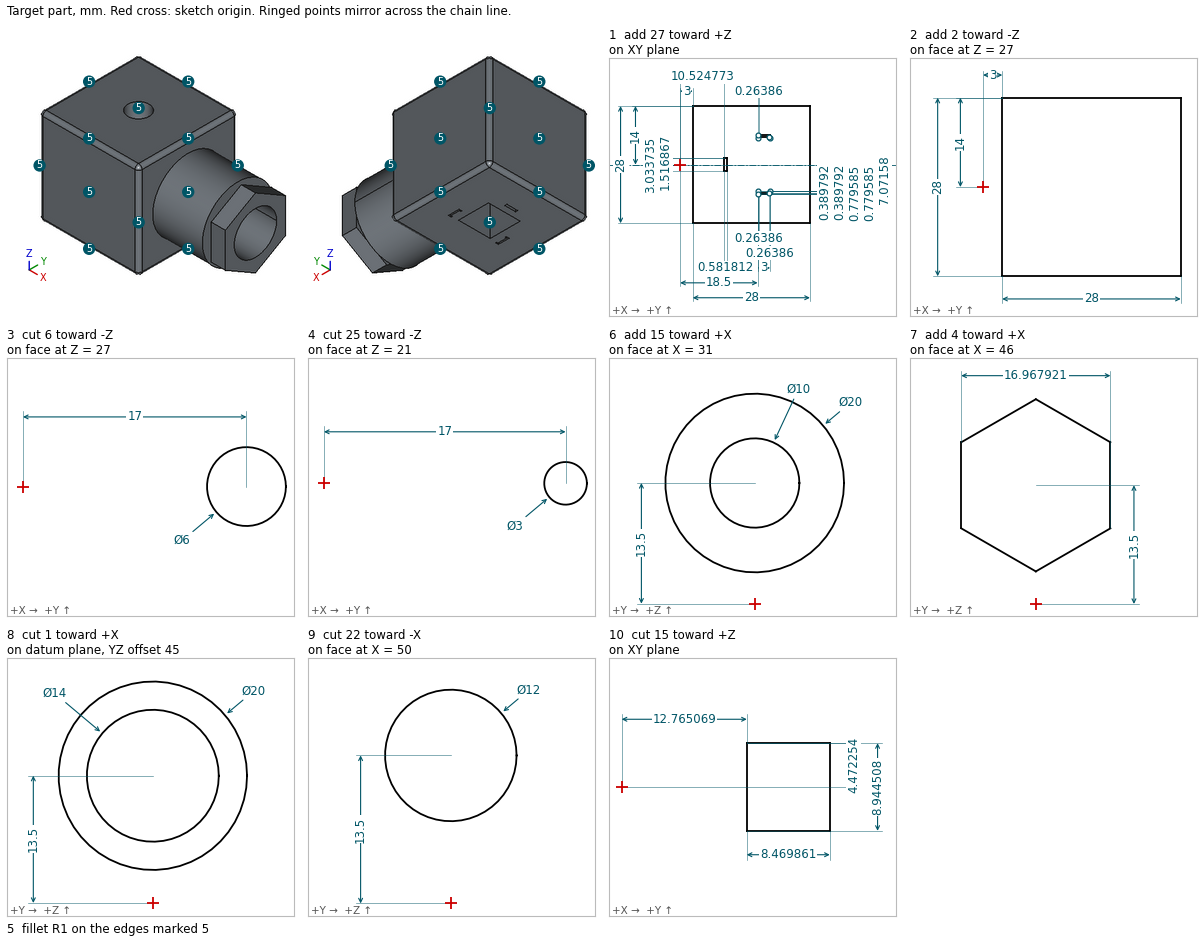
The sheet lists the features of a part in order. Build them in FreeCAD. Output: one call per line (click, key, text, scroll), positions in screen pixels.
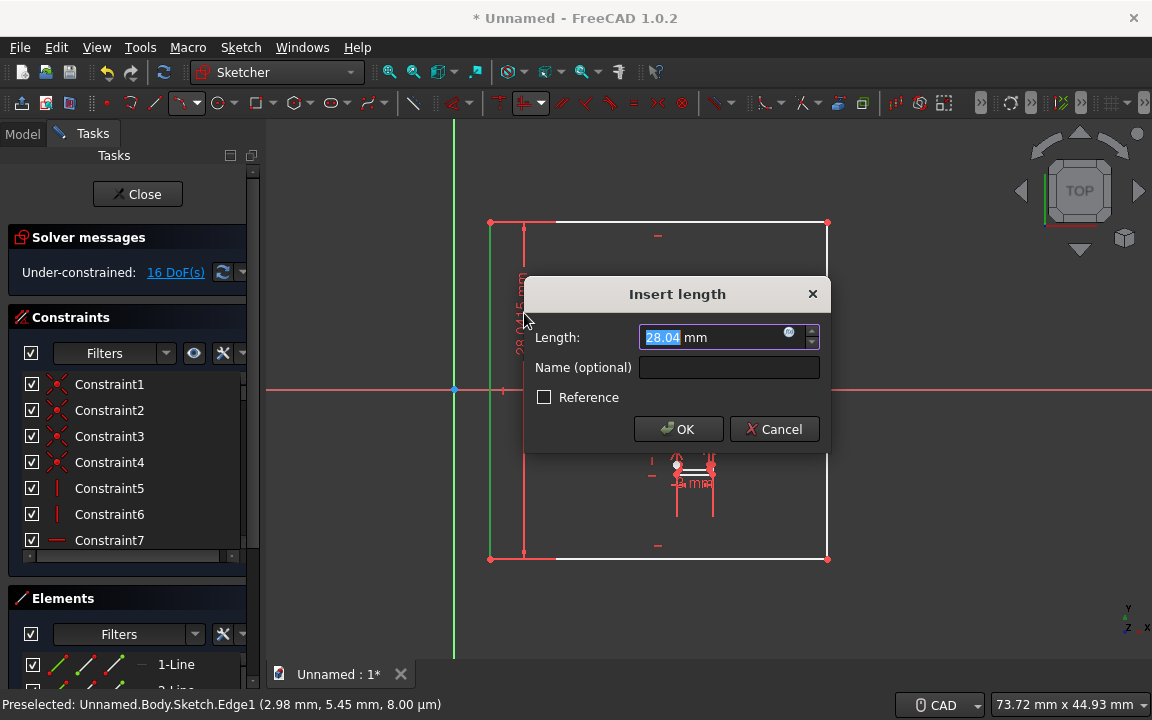
text(28)
key(Return)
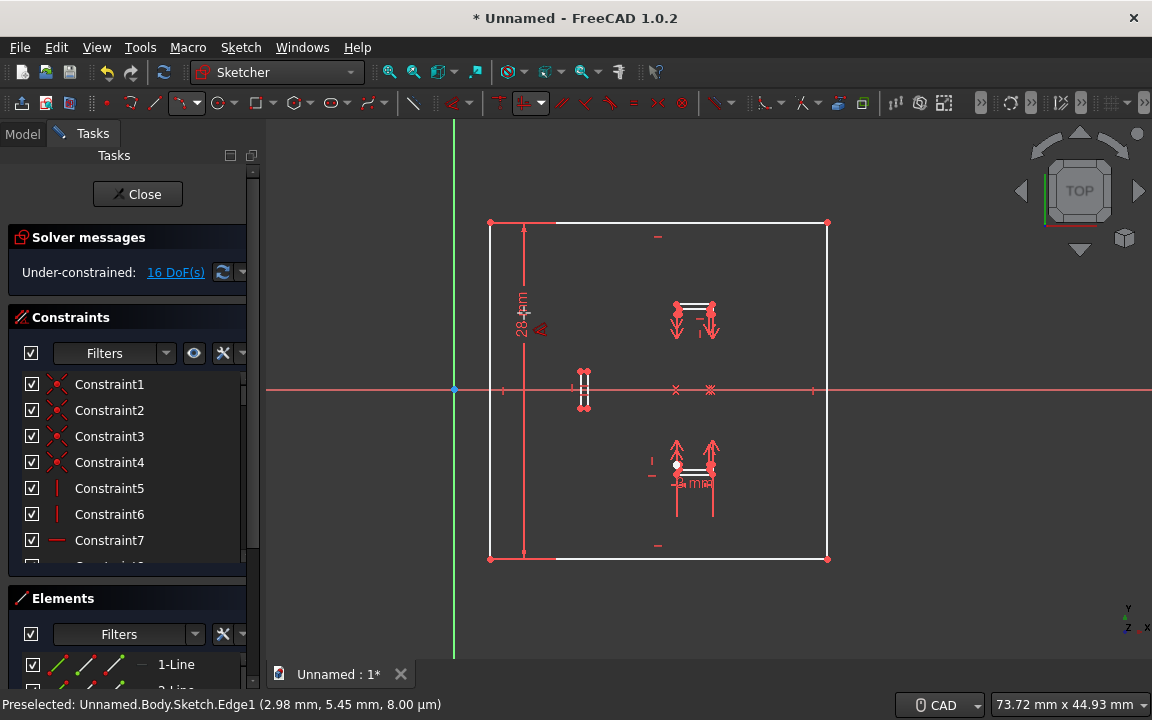
click(591, 559)
click(659, 593)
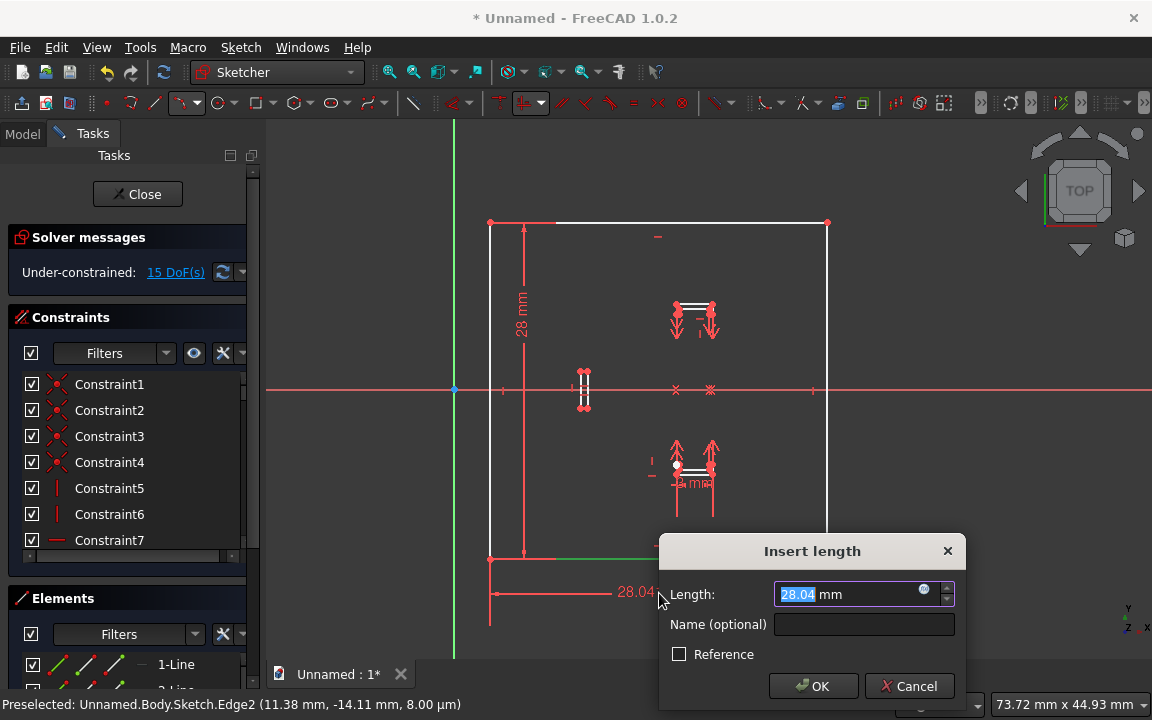
text(28)
key(Return)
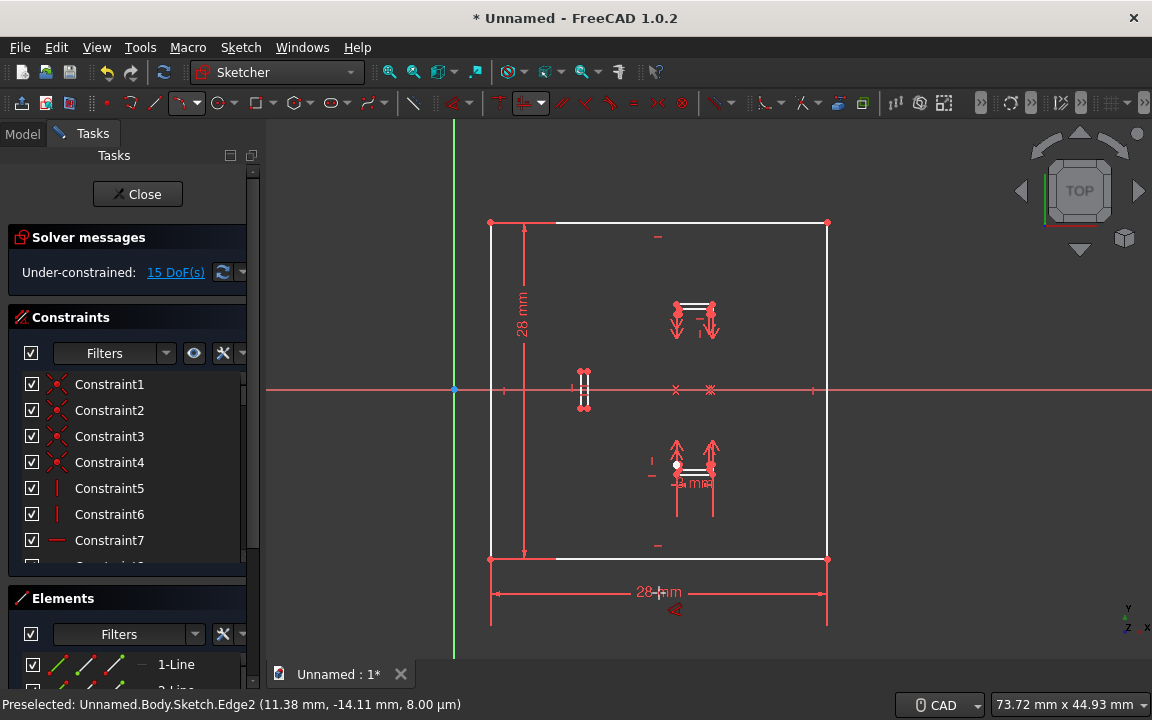
click(491, 223)
click(472, 189)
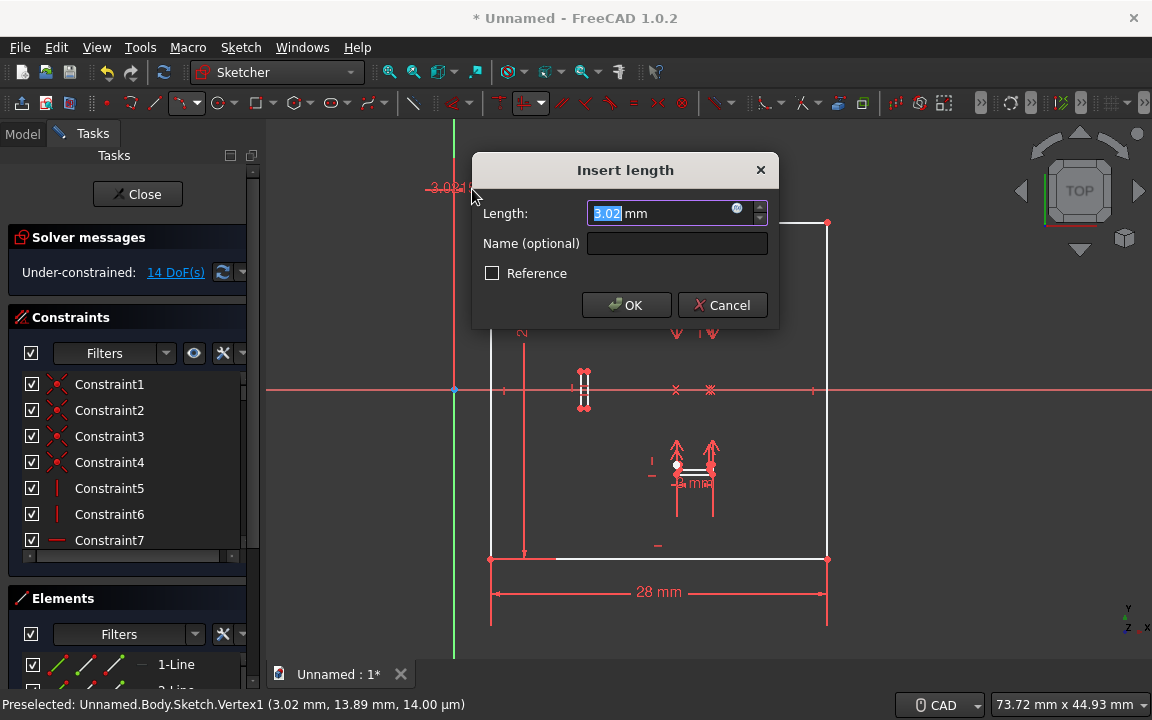
text(3)
key(Return)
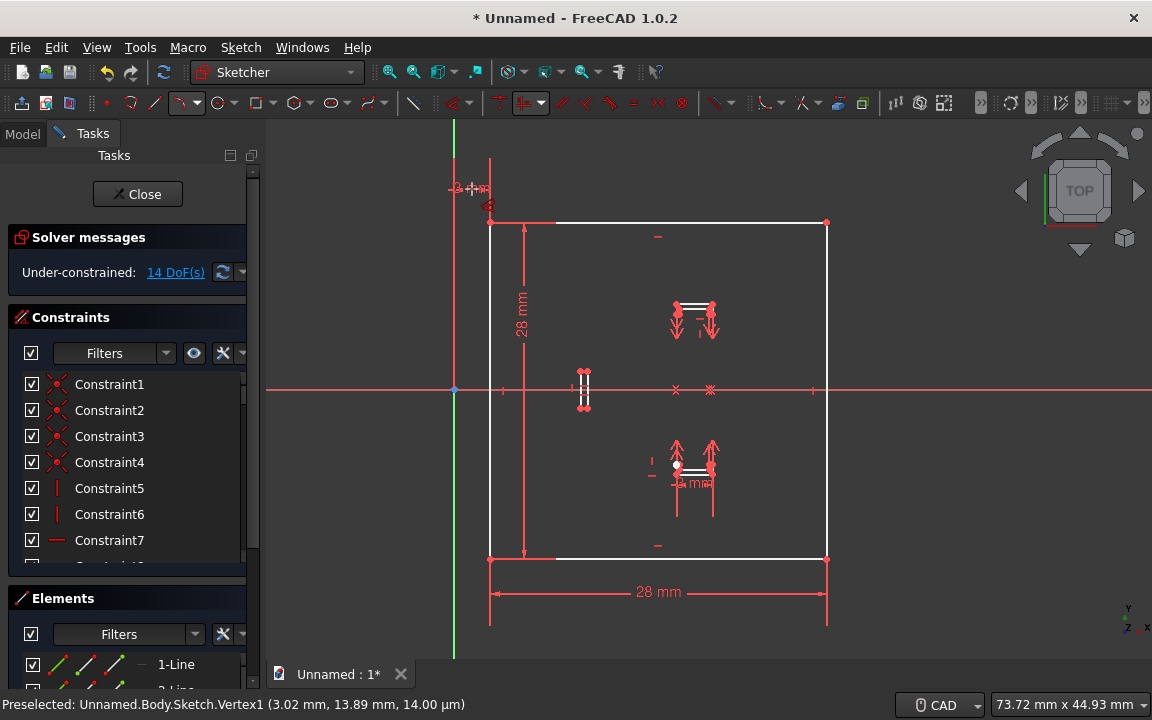
click(490, 223)
click(420, 306)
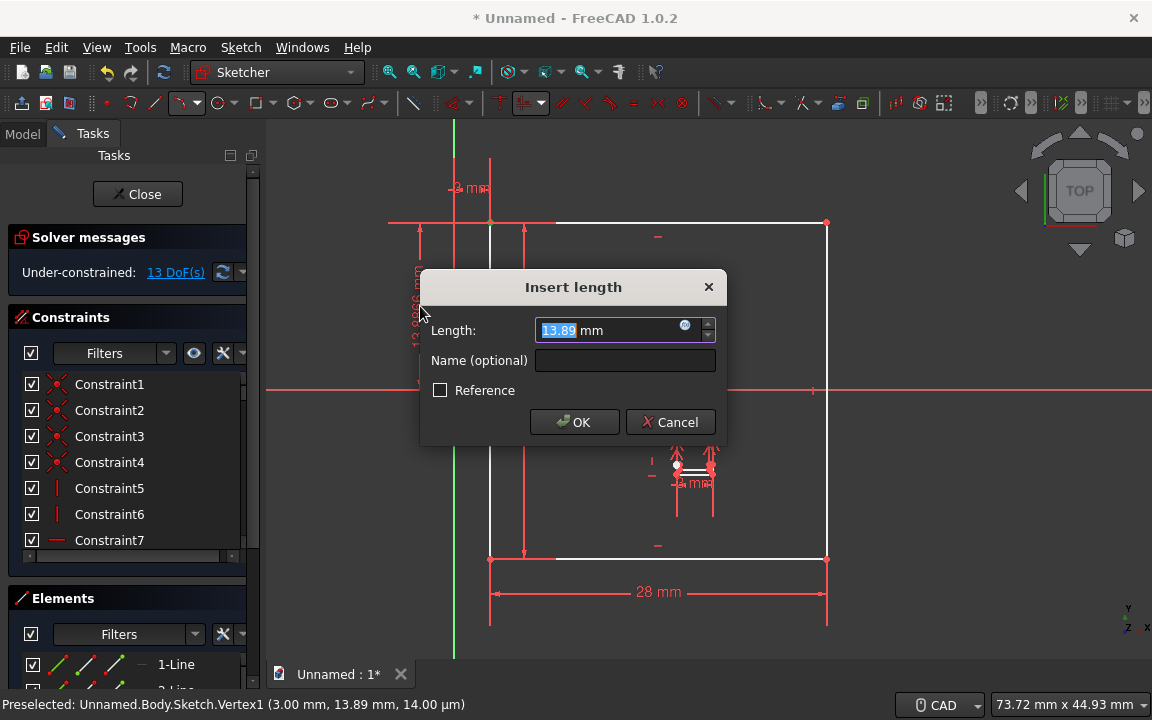
text(14)
key(Return)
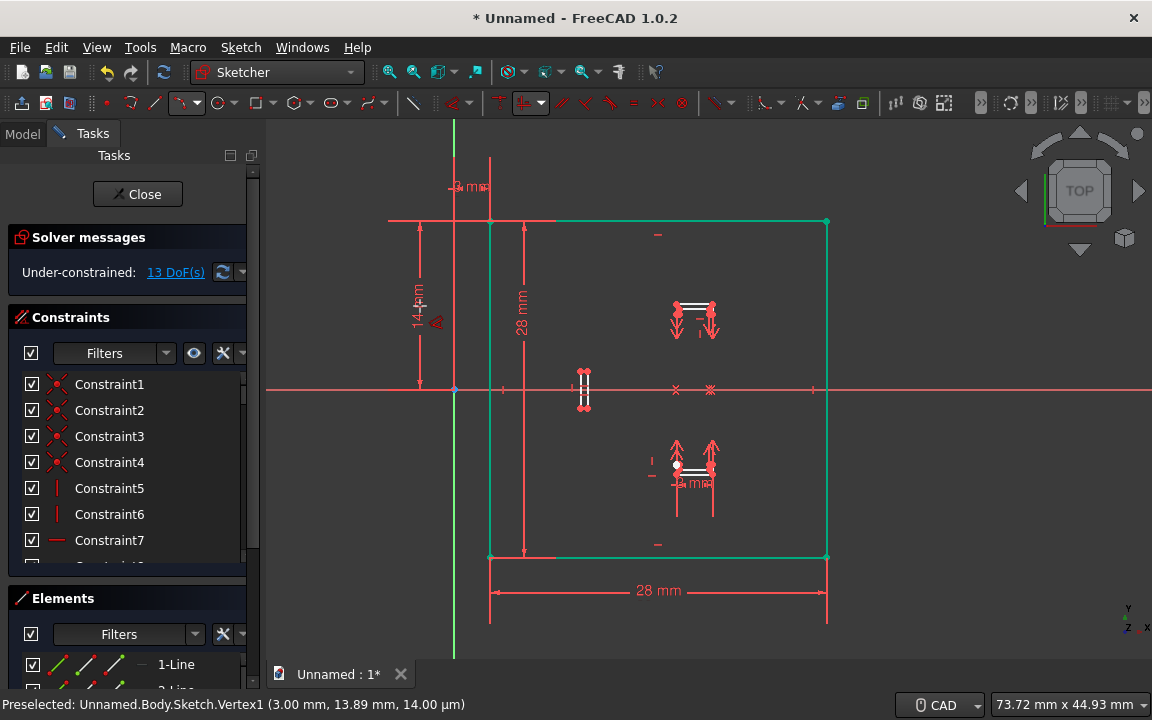
scroll(677, 465, up, 7)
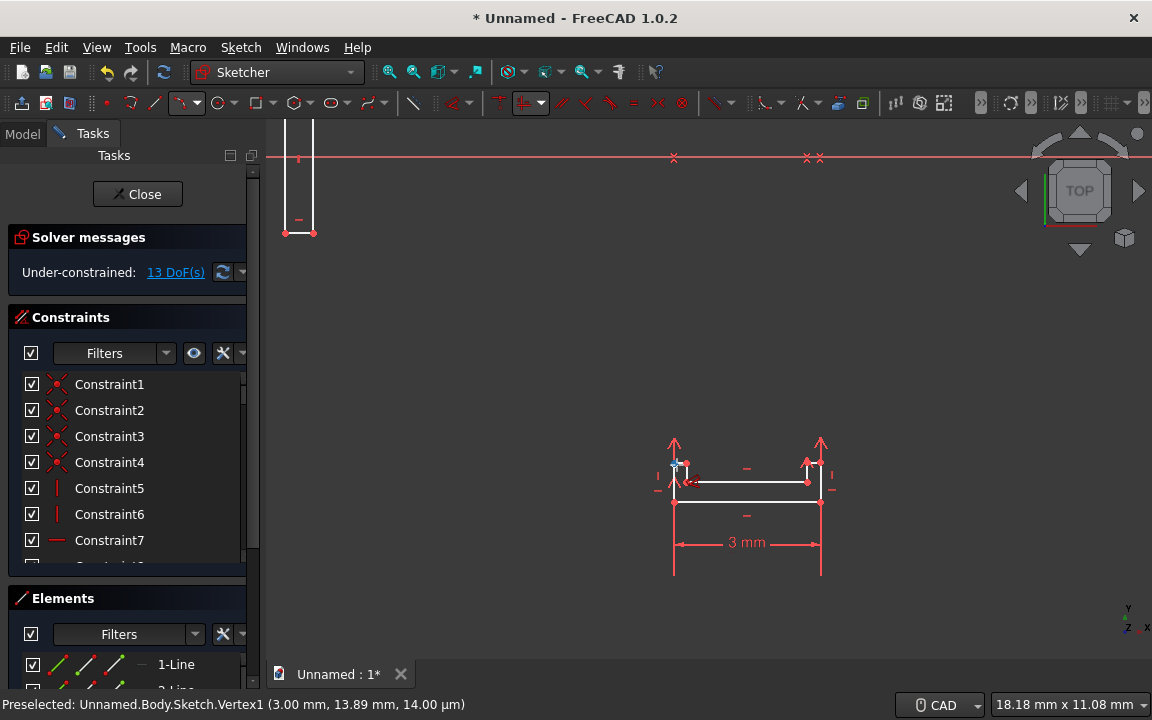
click(674, 463)
click(484, 497)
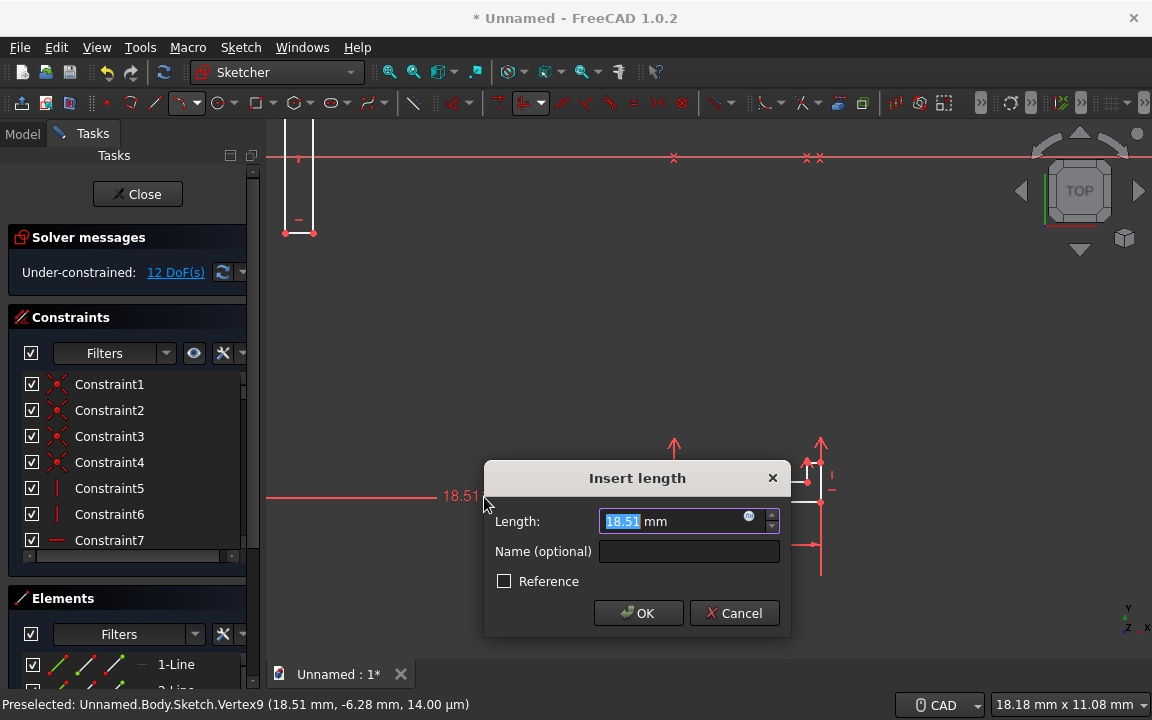
text(18.5)
key(Return)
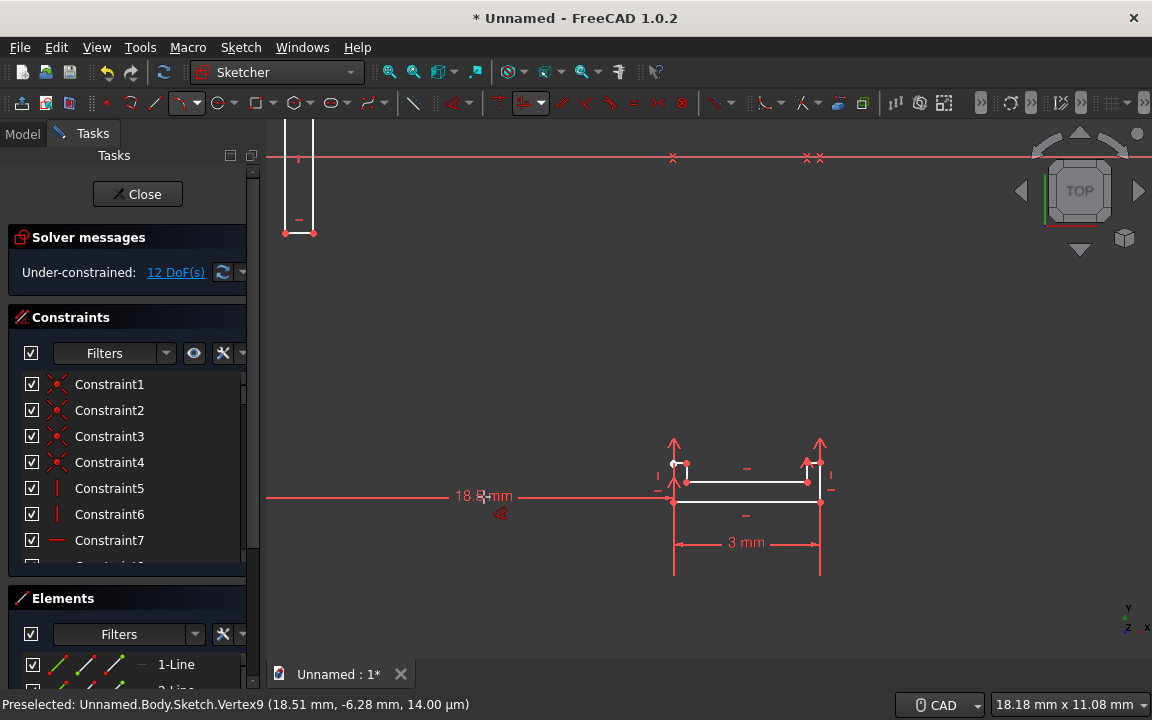
scroll(680, 463, up, 6)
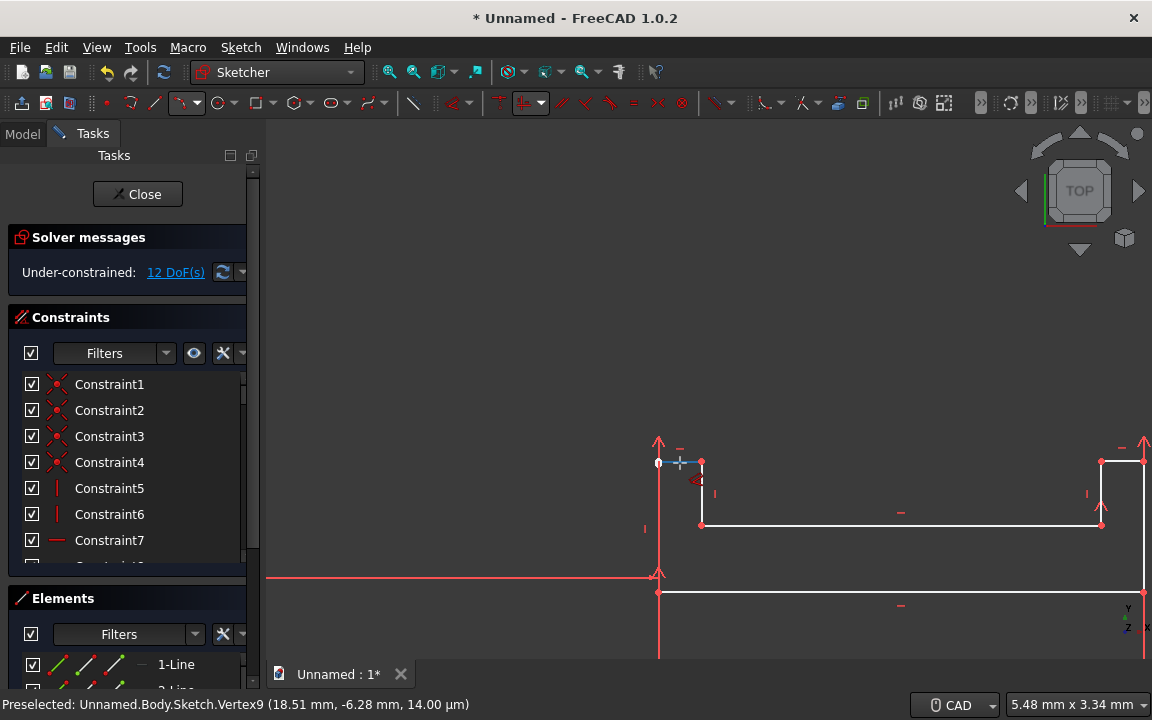
click(680, 462)
click(680, 496)